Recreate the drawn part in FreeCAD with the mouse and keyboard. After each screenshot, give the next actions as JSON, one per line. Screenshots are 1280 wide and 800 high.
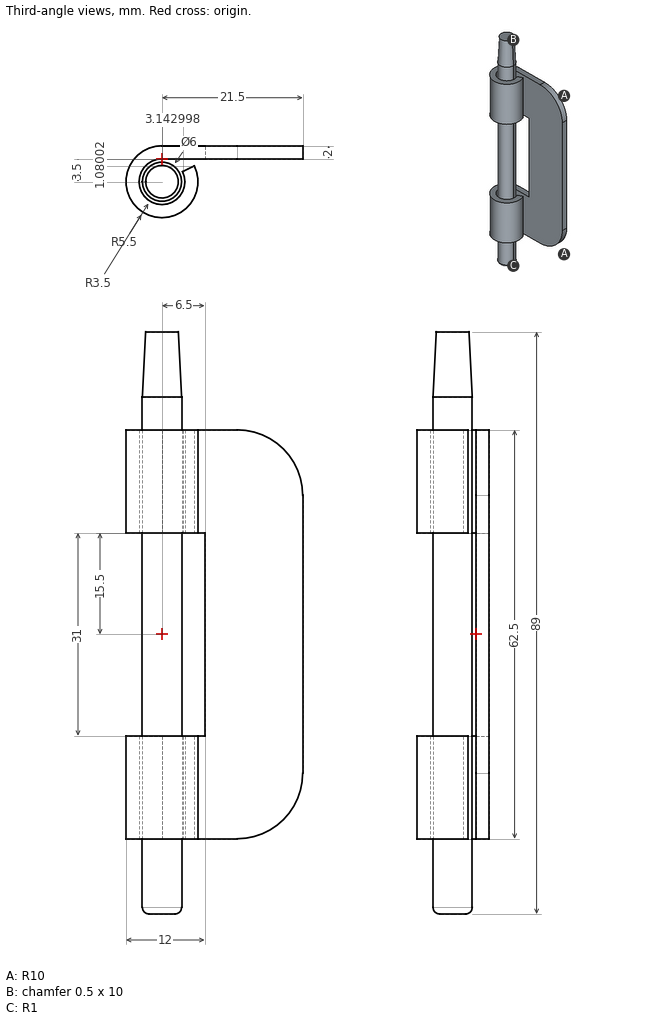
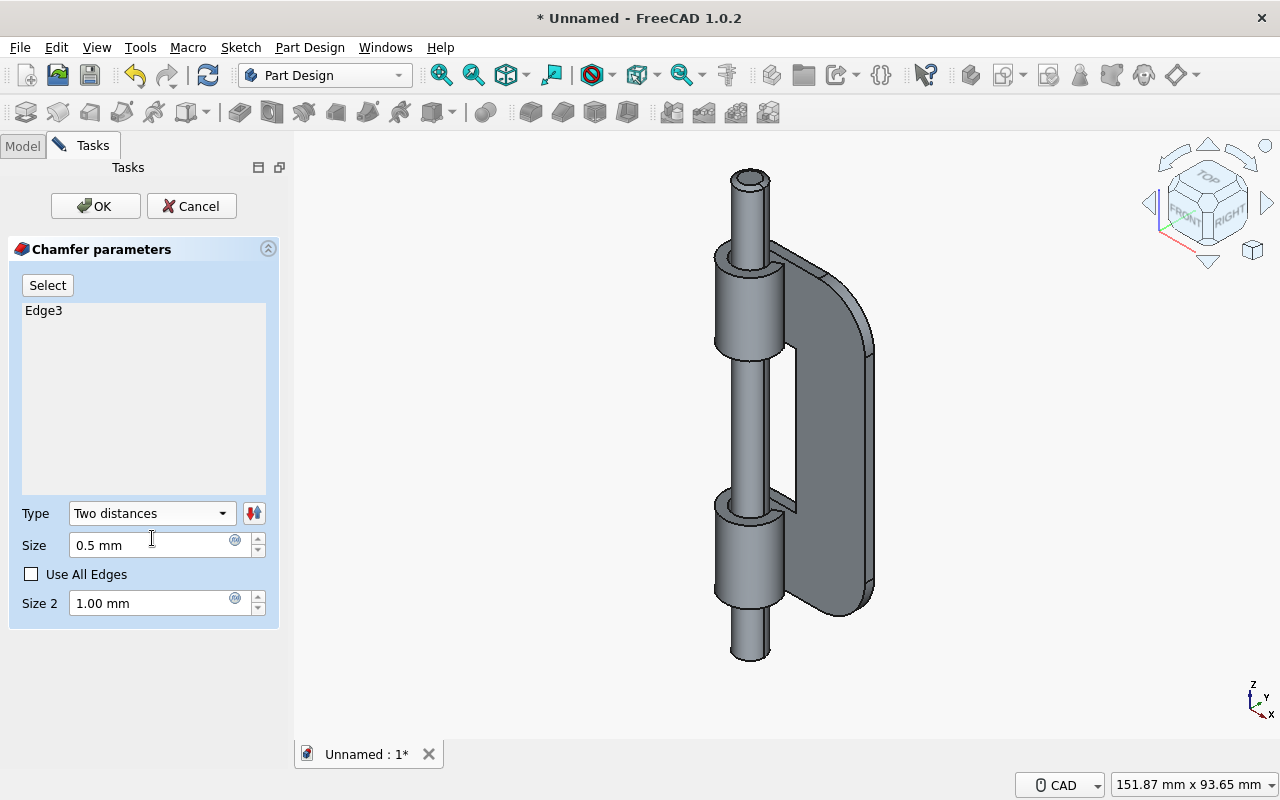
{"action": "triple_click", "coordinate": [160, 603]}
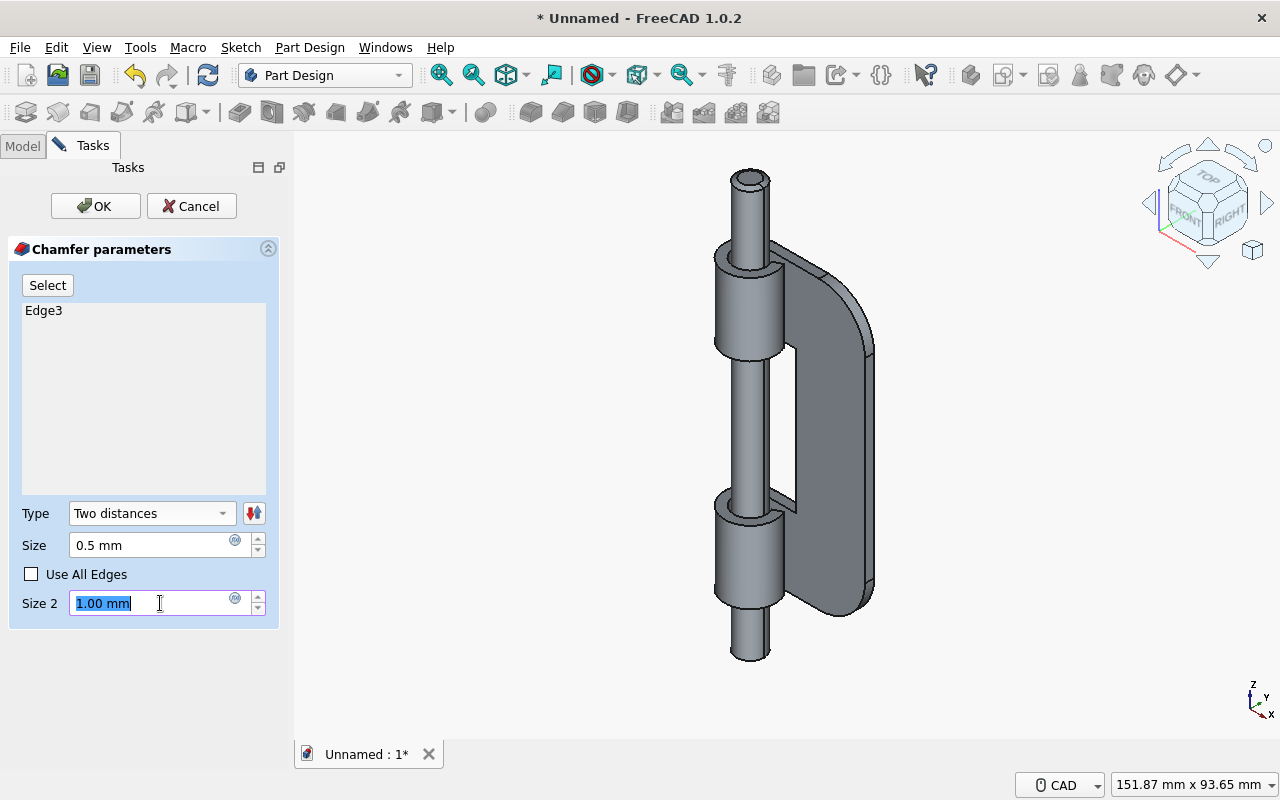
{"action": "type", "text": "10"}
{"action": "key", "text": "Tab"}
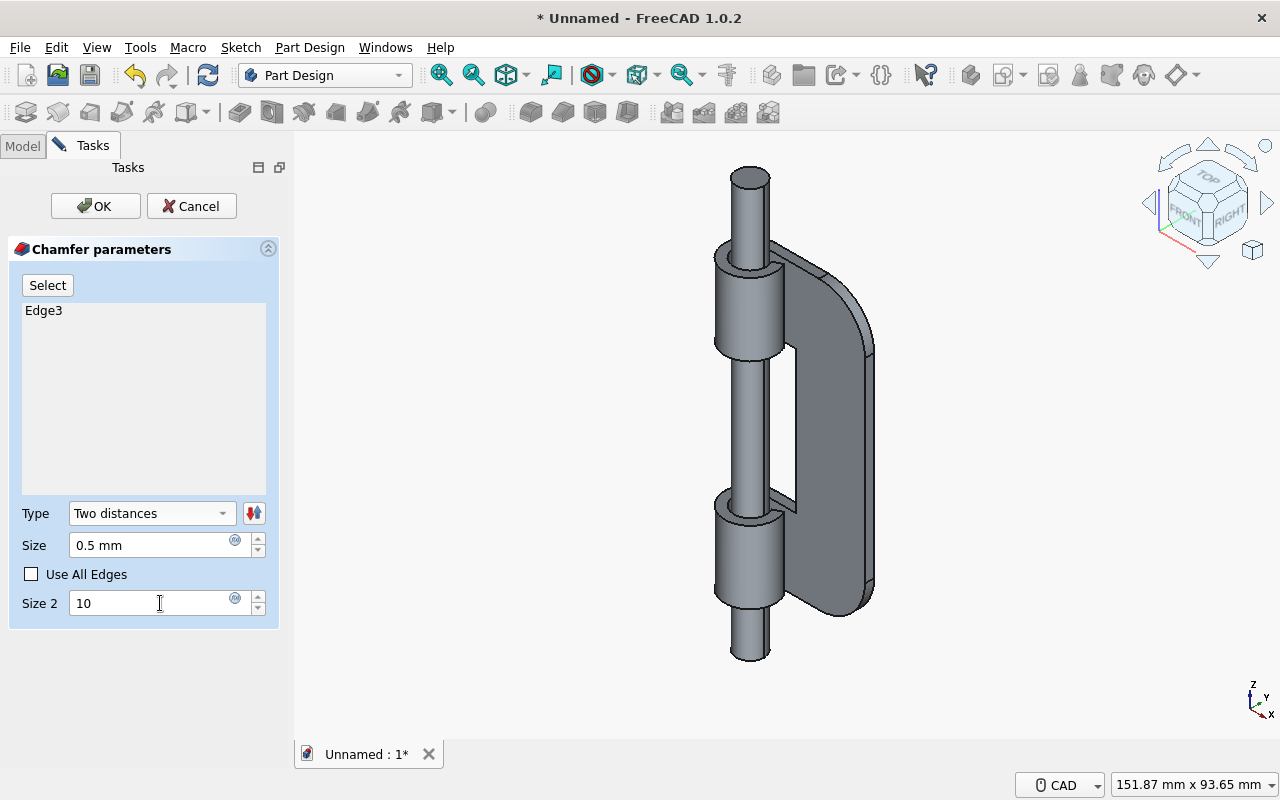
{"action": "left_click", "coordinate": [254, 514]}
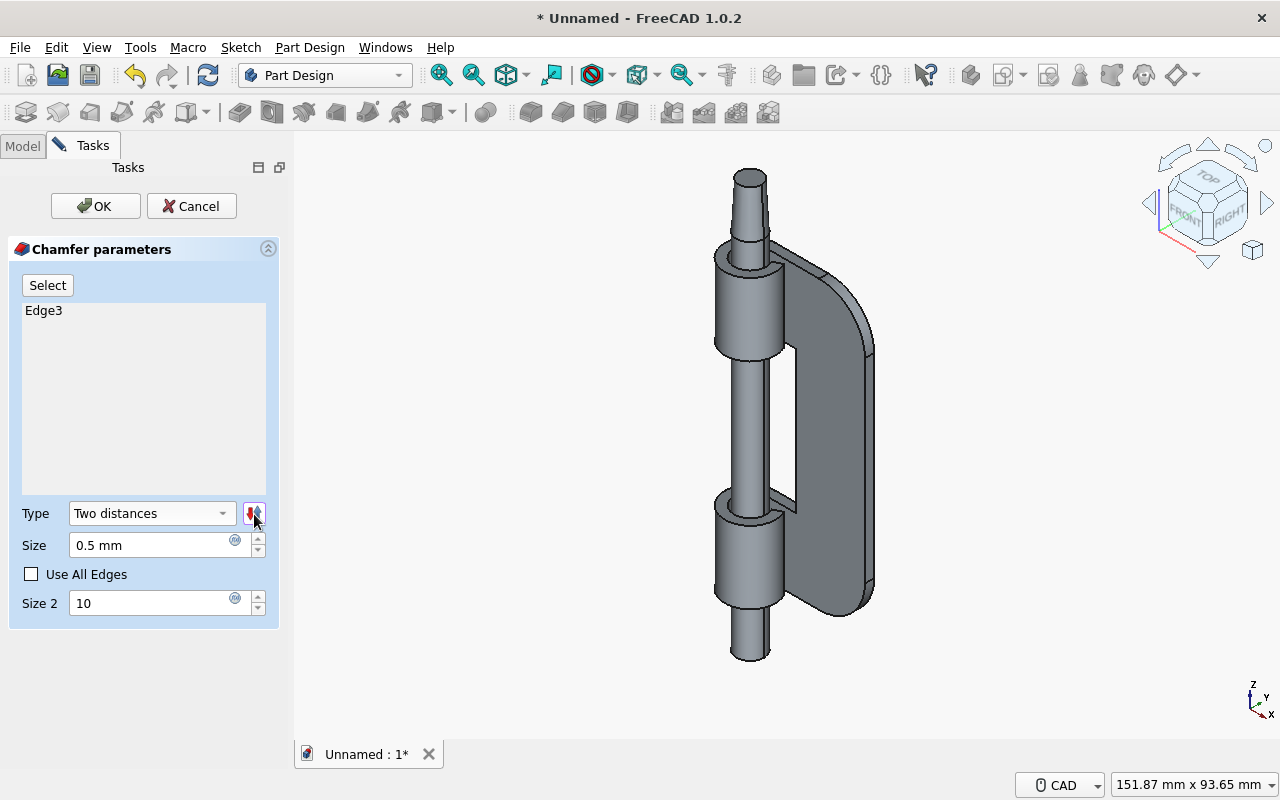
{"action": "left_click", "coordinate": [96, 206]}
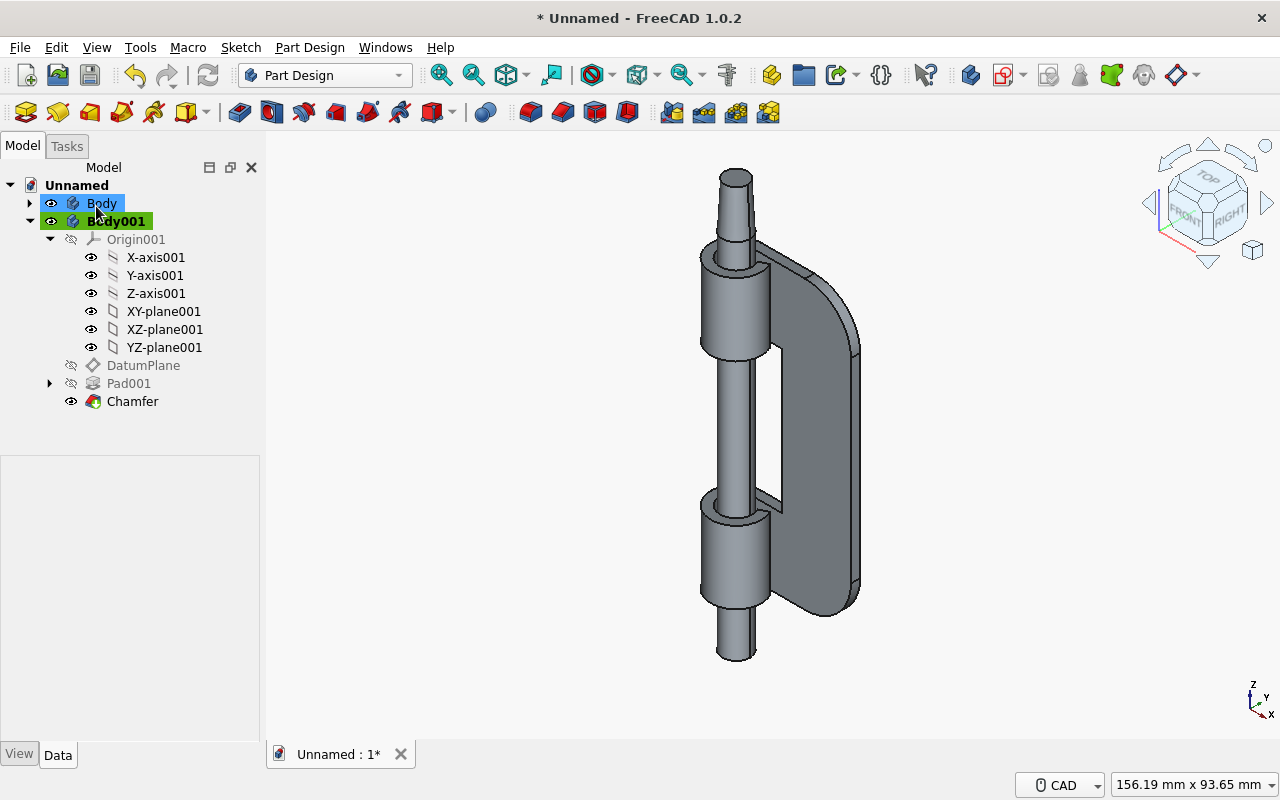
{"action": "key", "text": "2"}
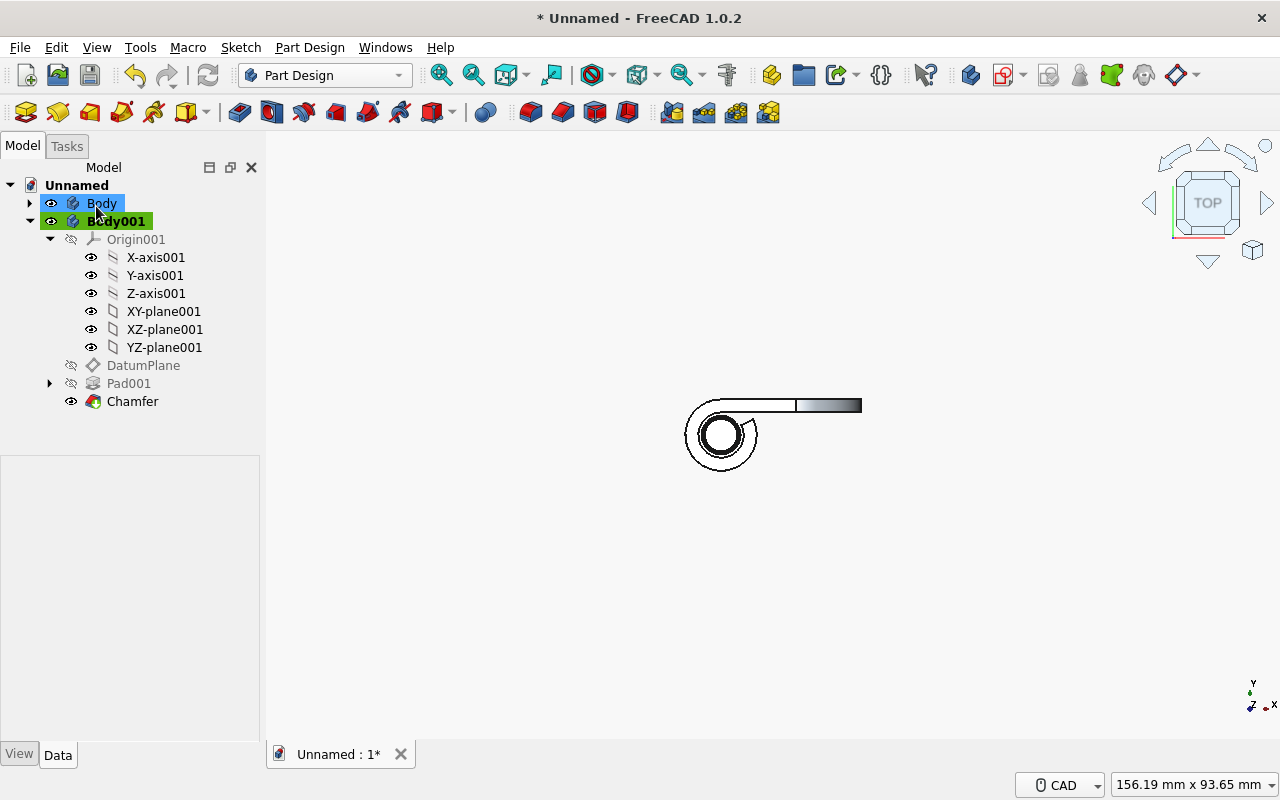
{"action": "key", "text": "v f"}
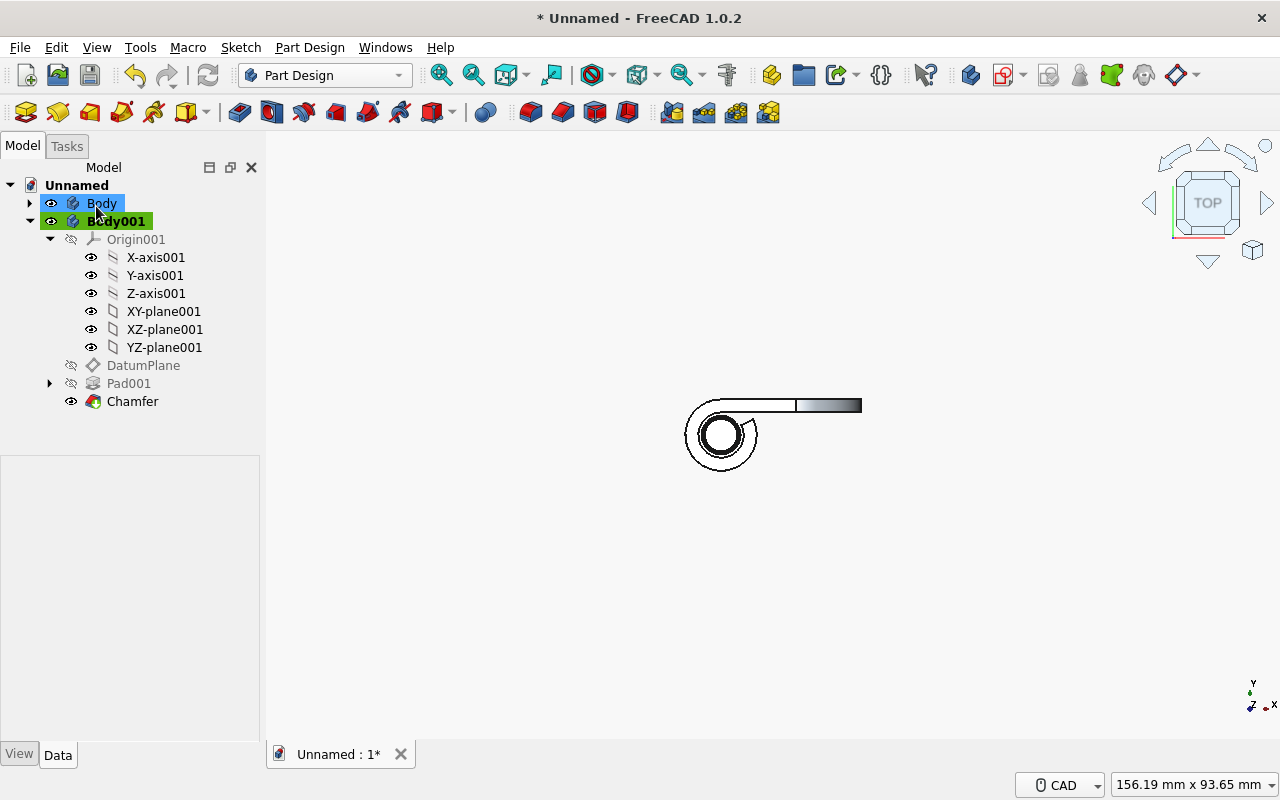
{"action": "key", "text": "0"}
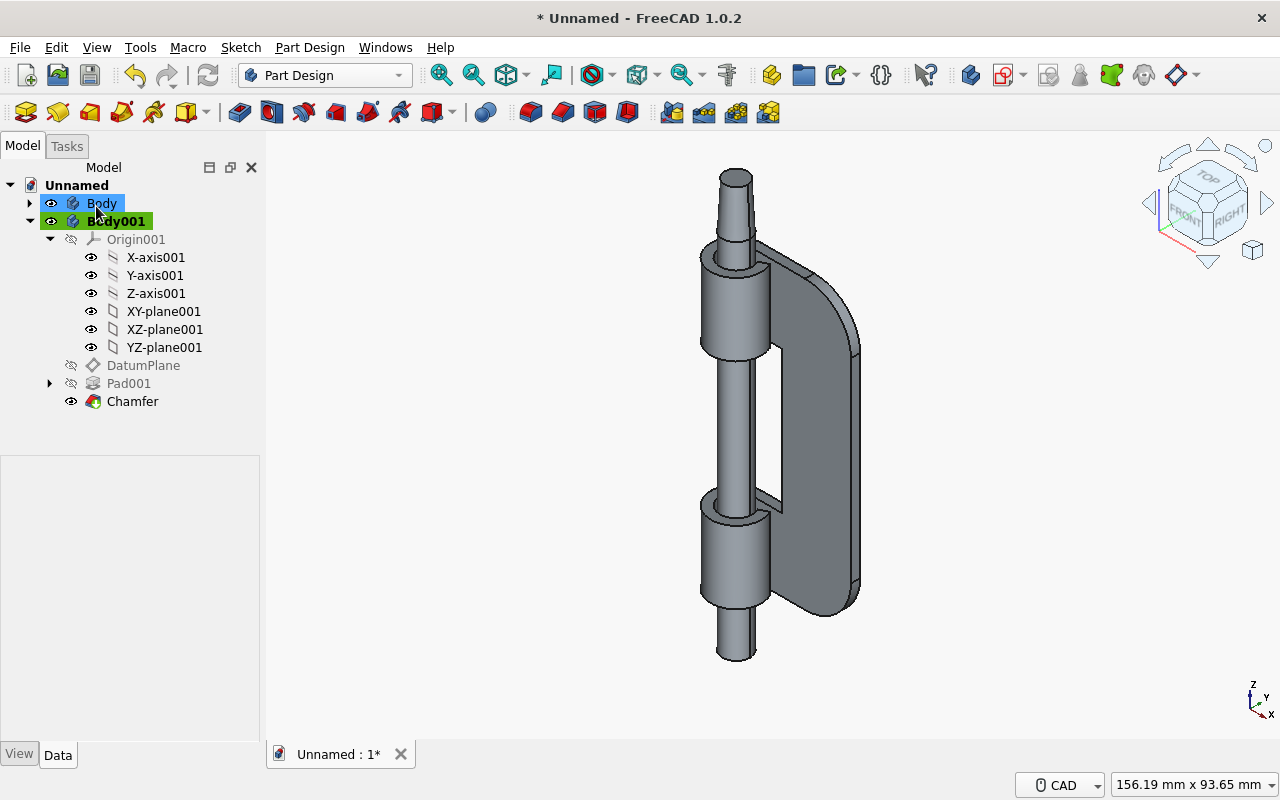
{"action": "key", "text": "1"}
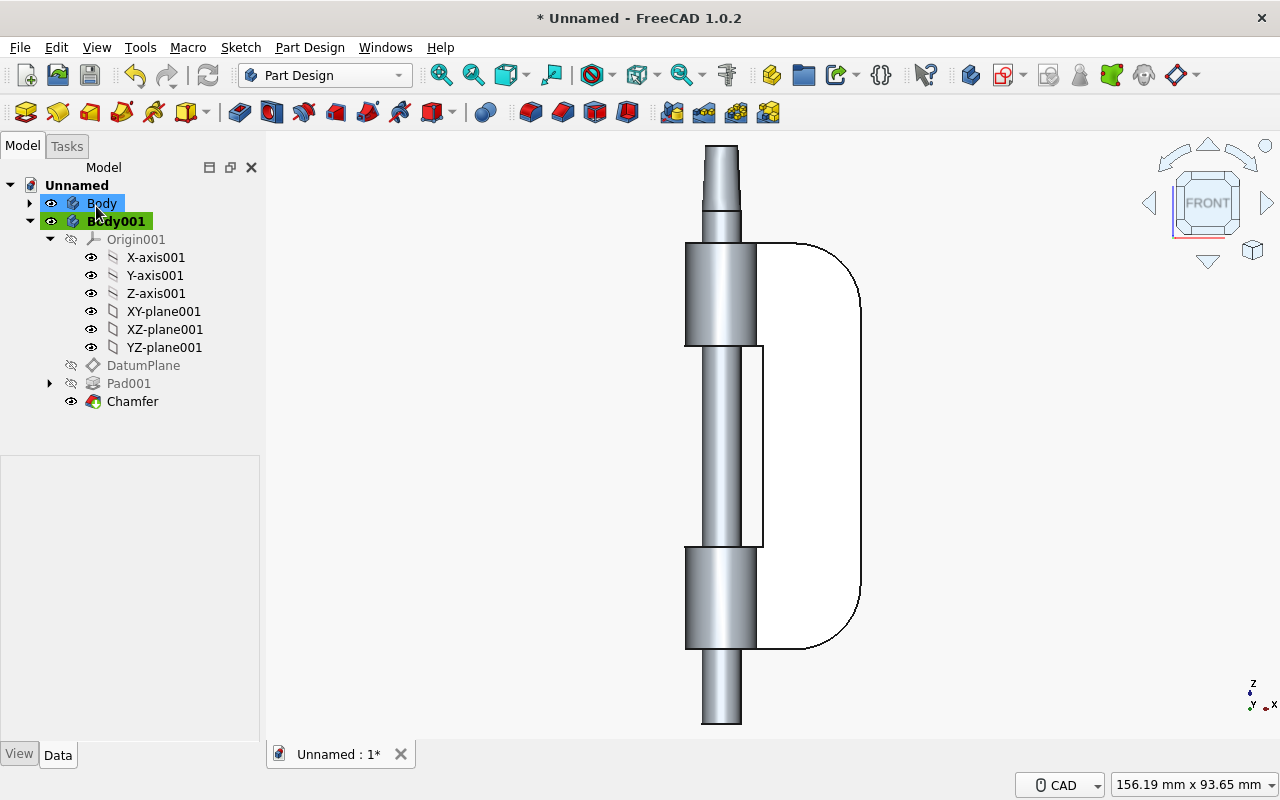
{"action": "key", "text": "3"}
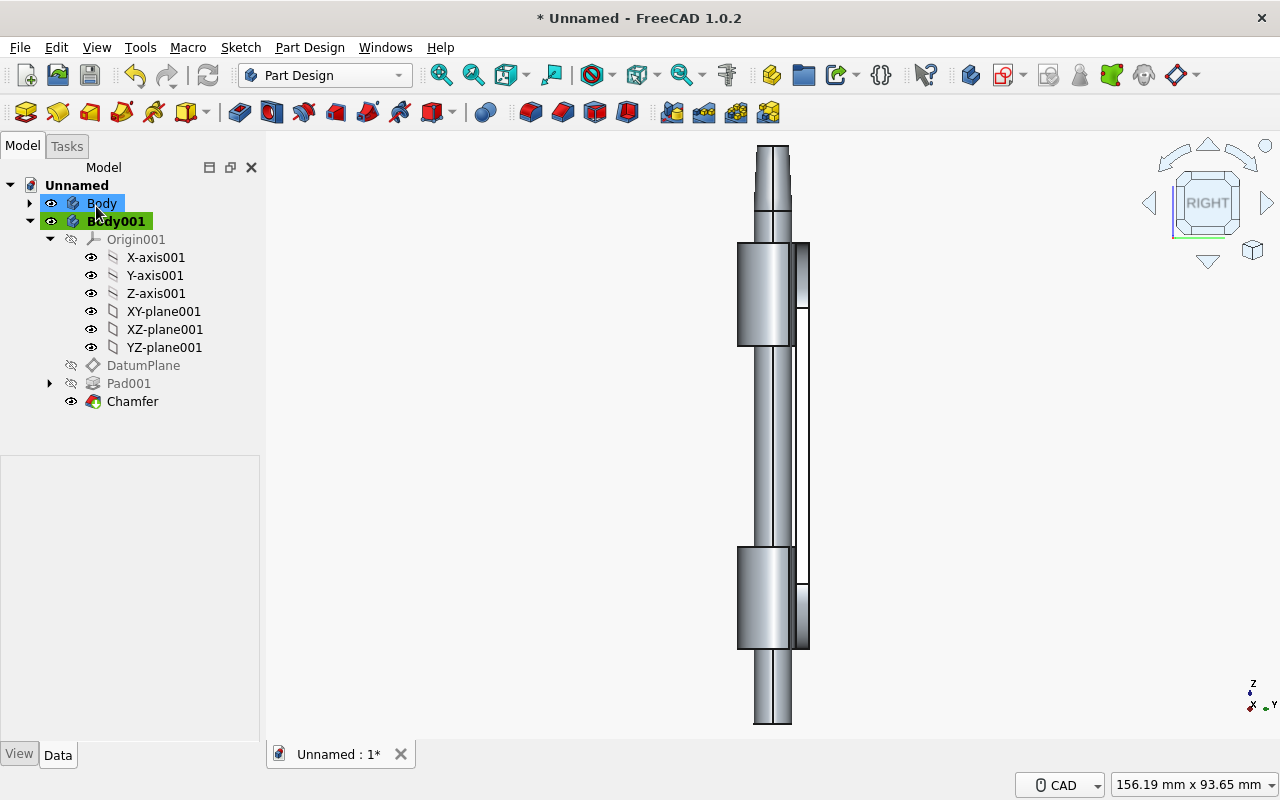
{"action": "key", "text": "5"}